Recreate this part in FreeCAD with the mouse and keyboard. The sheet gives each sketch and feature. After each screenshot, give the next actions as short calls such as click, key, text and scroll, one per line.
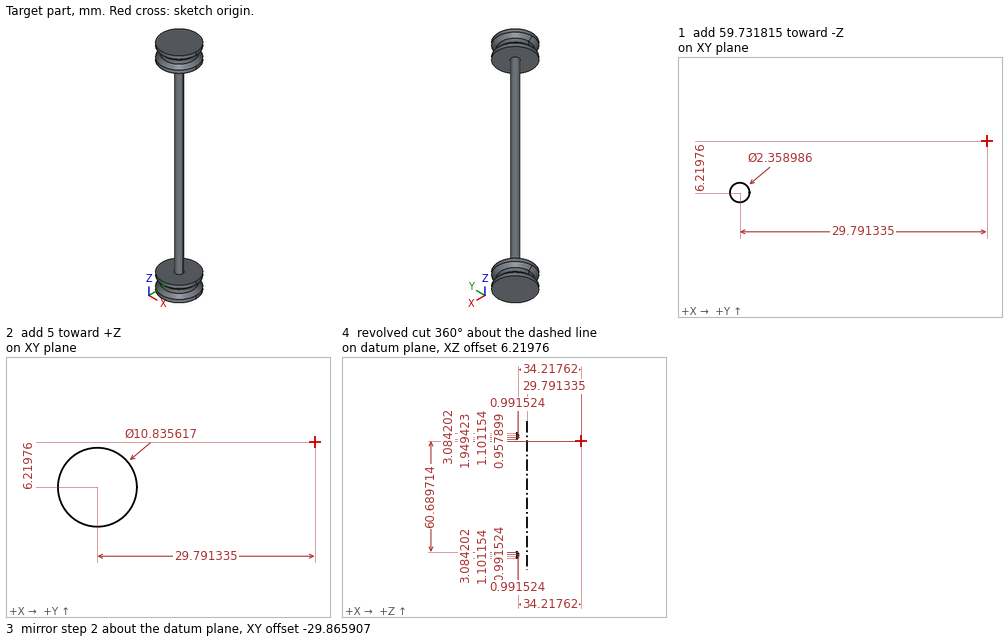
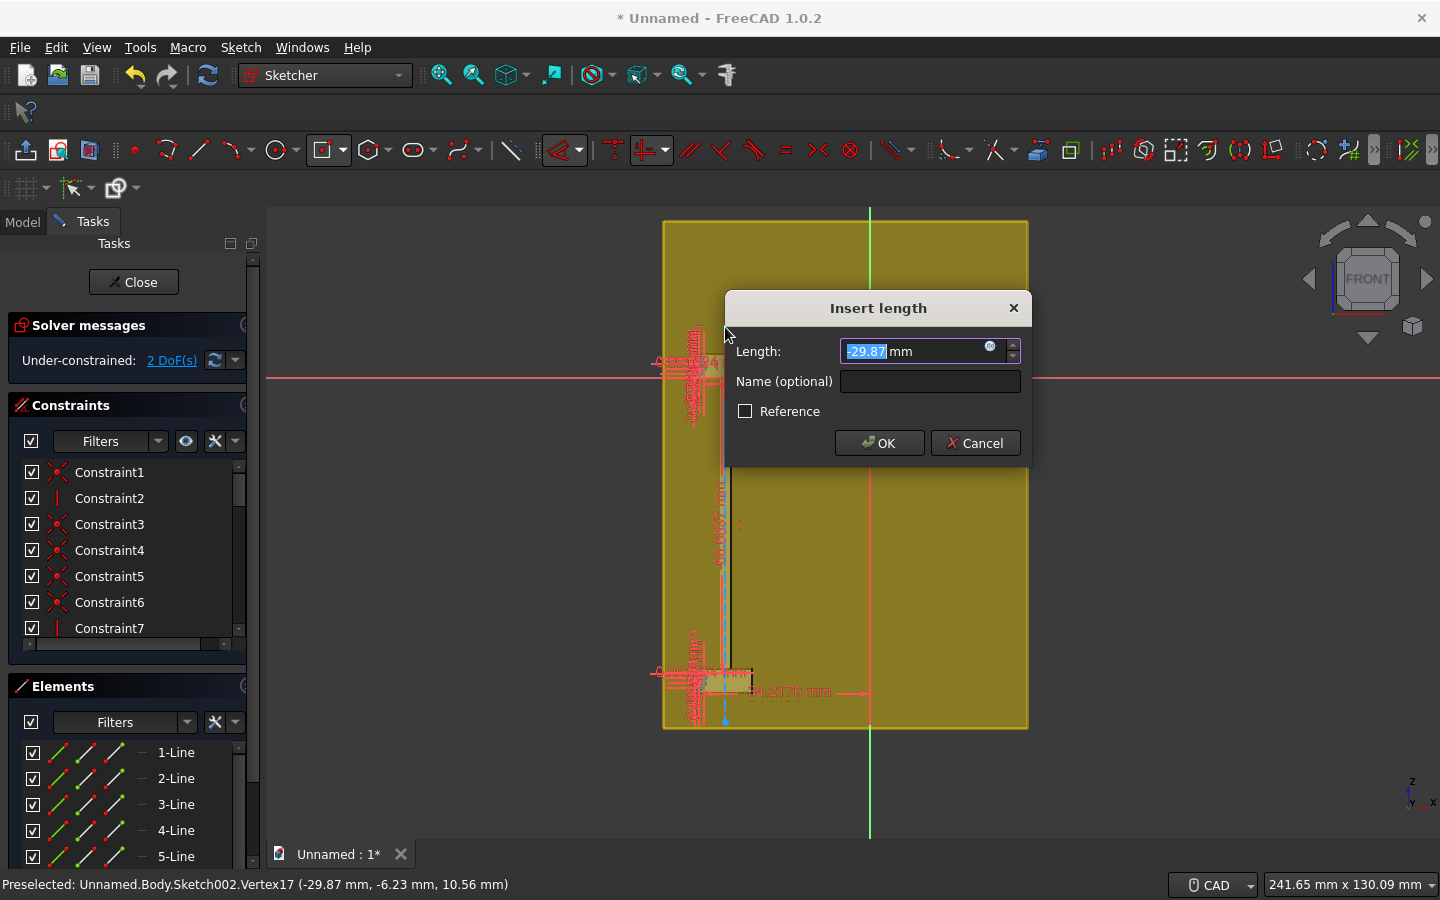
text(-29.791335)
key(Return)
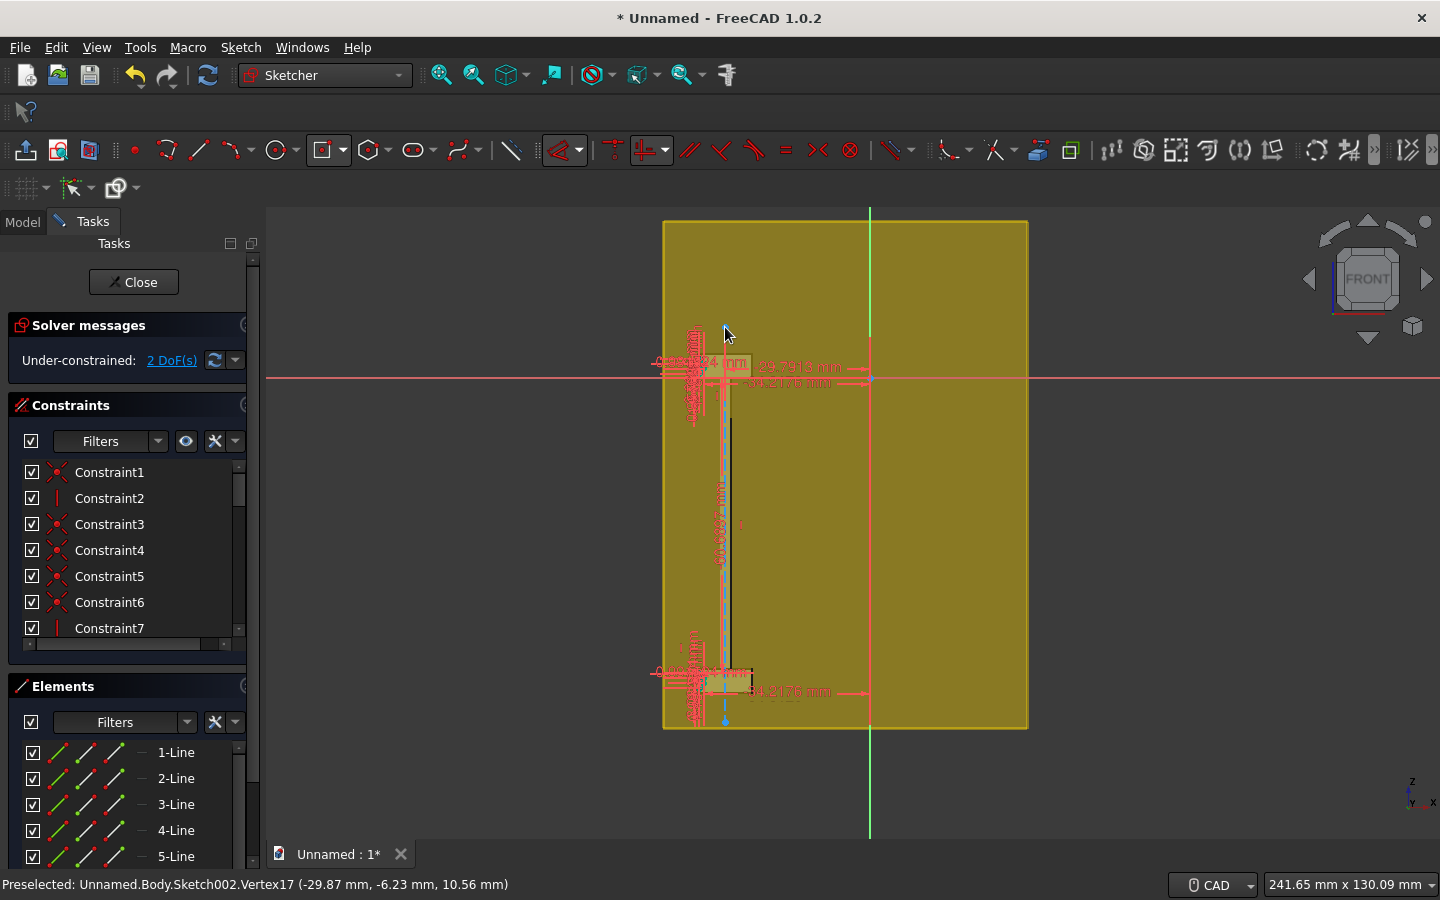
click(134, 282)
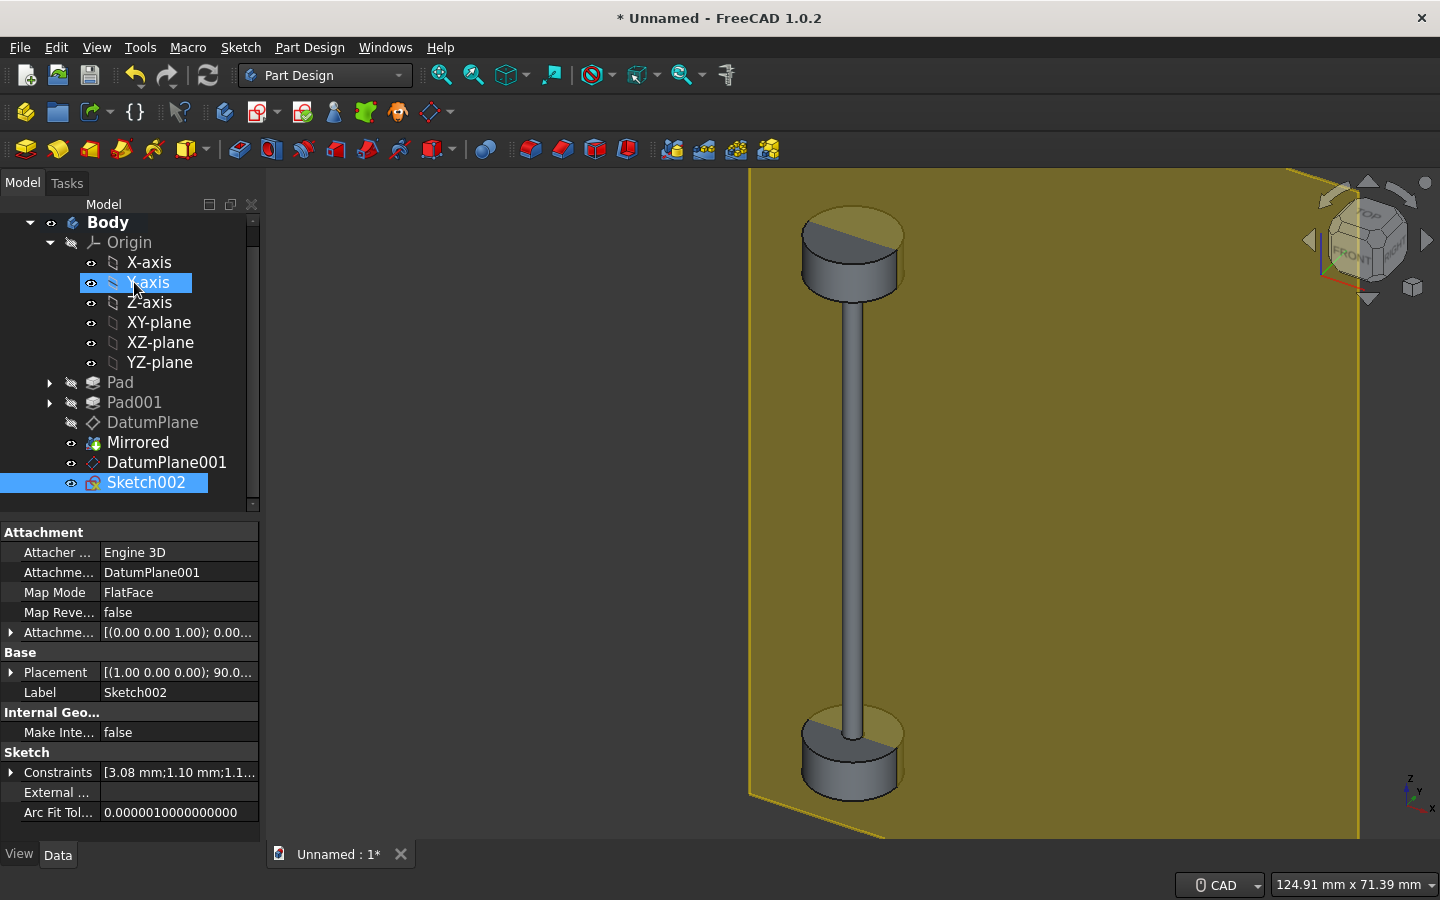
click(304, 150)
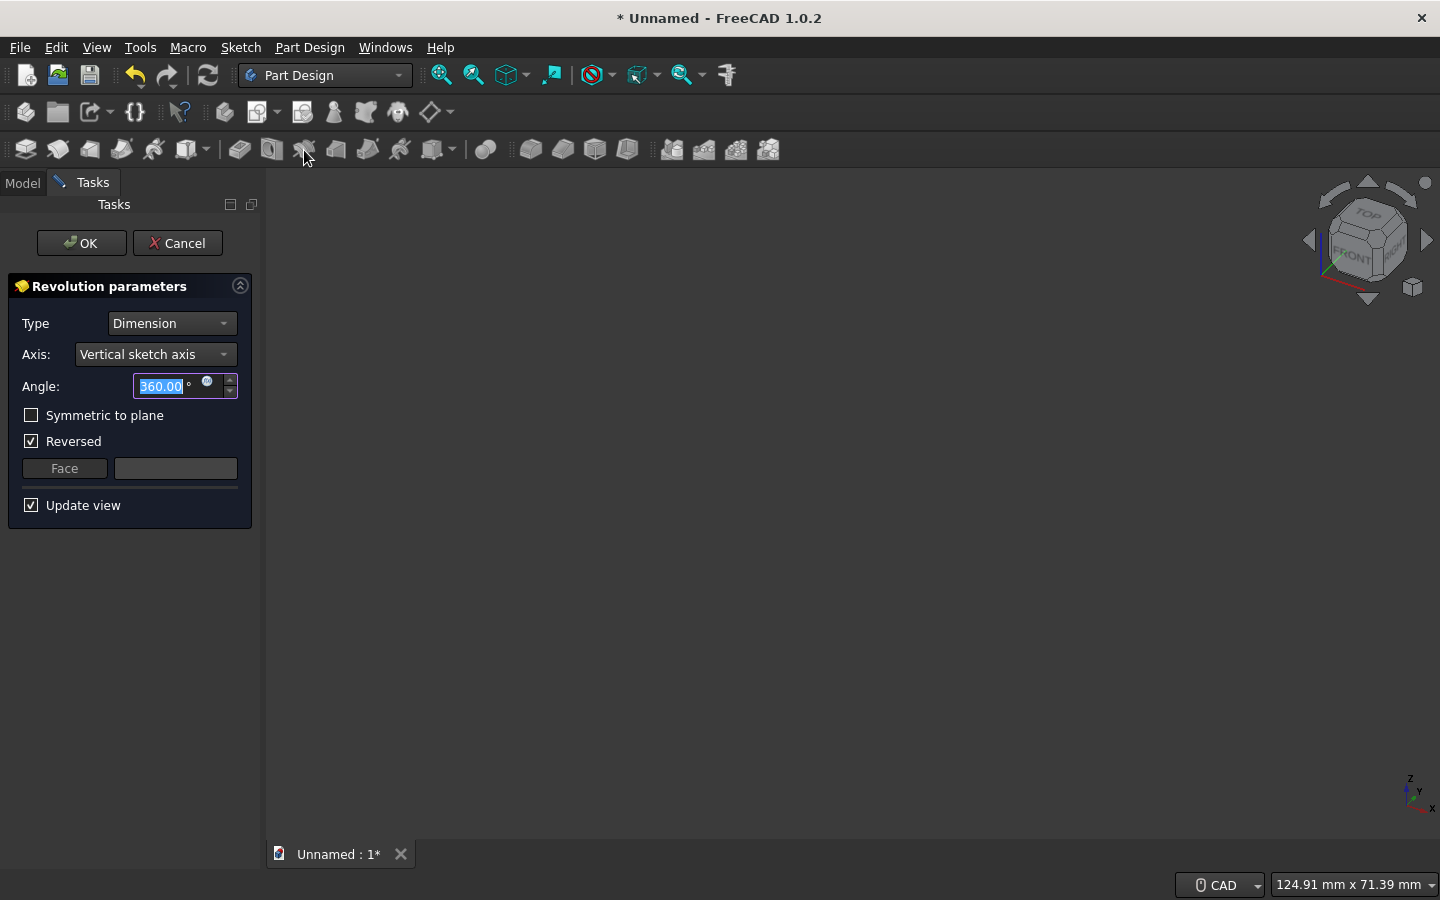
click(156, 354)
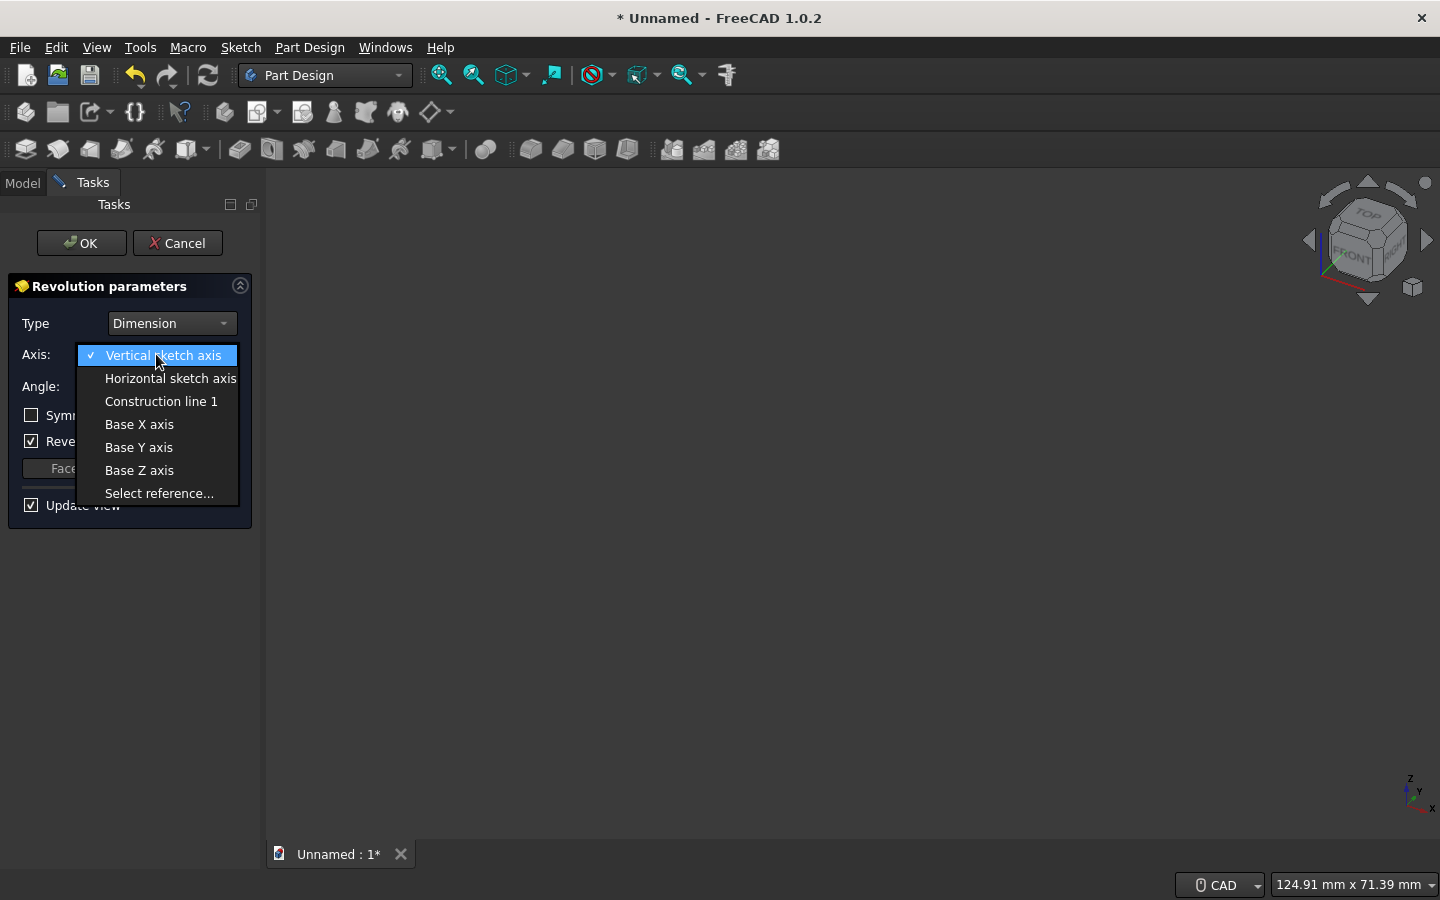
click(156, 402)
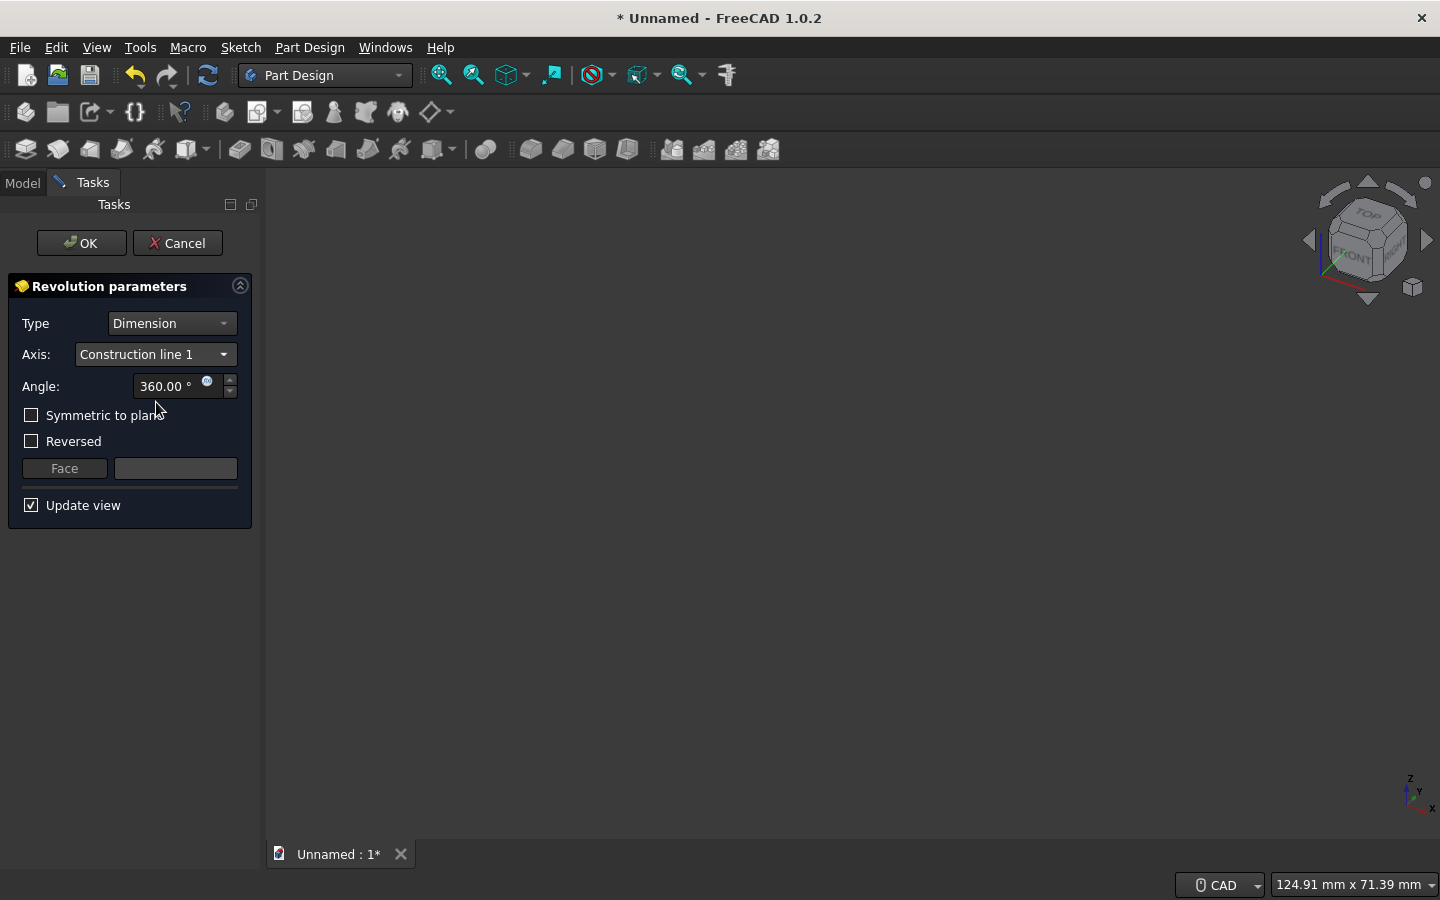
click(82, 243)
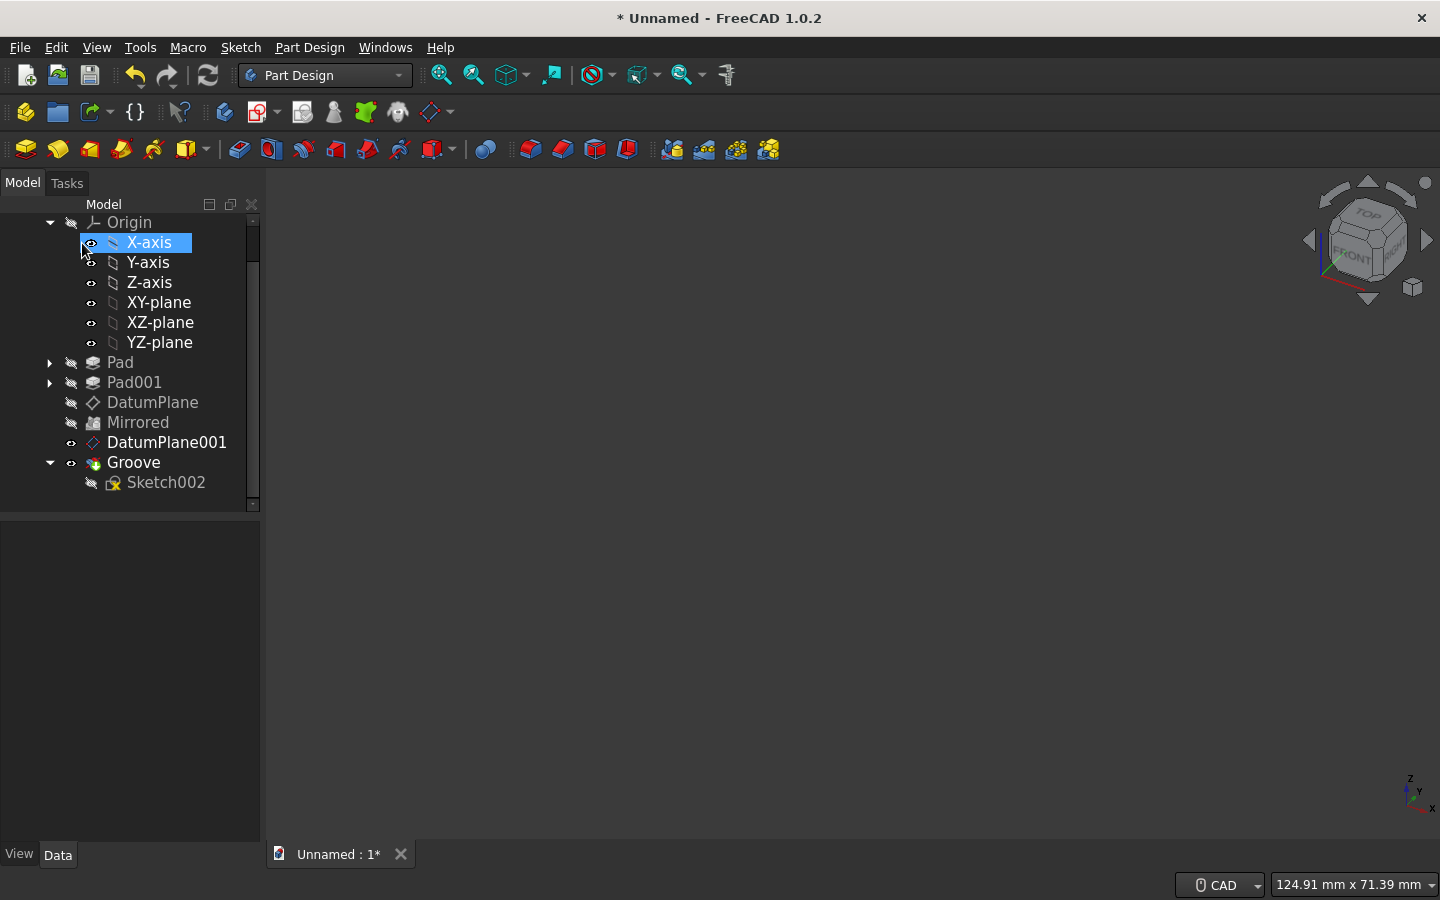
click(116, 443)
key(space)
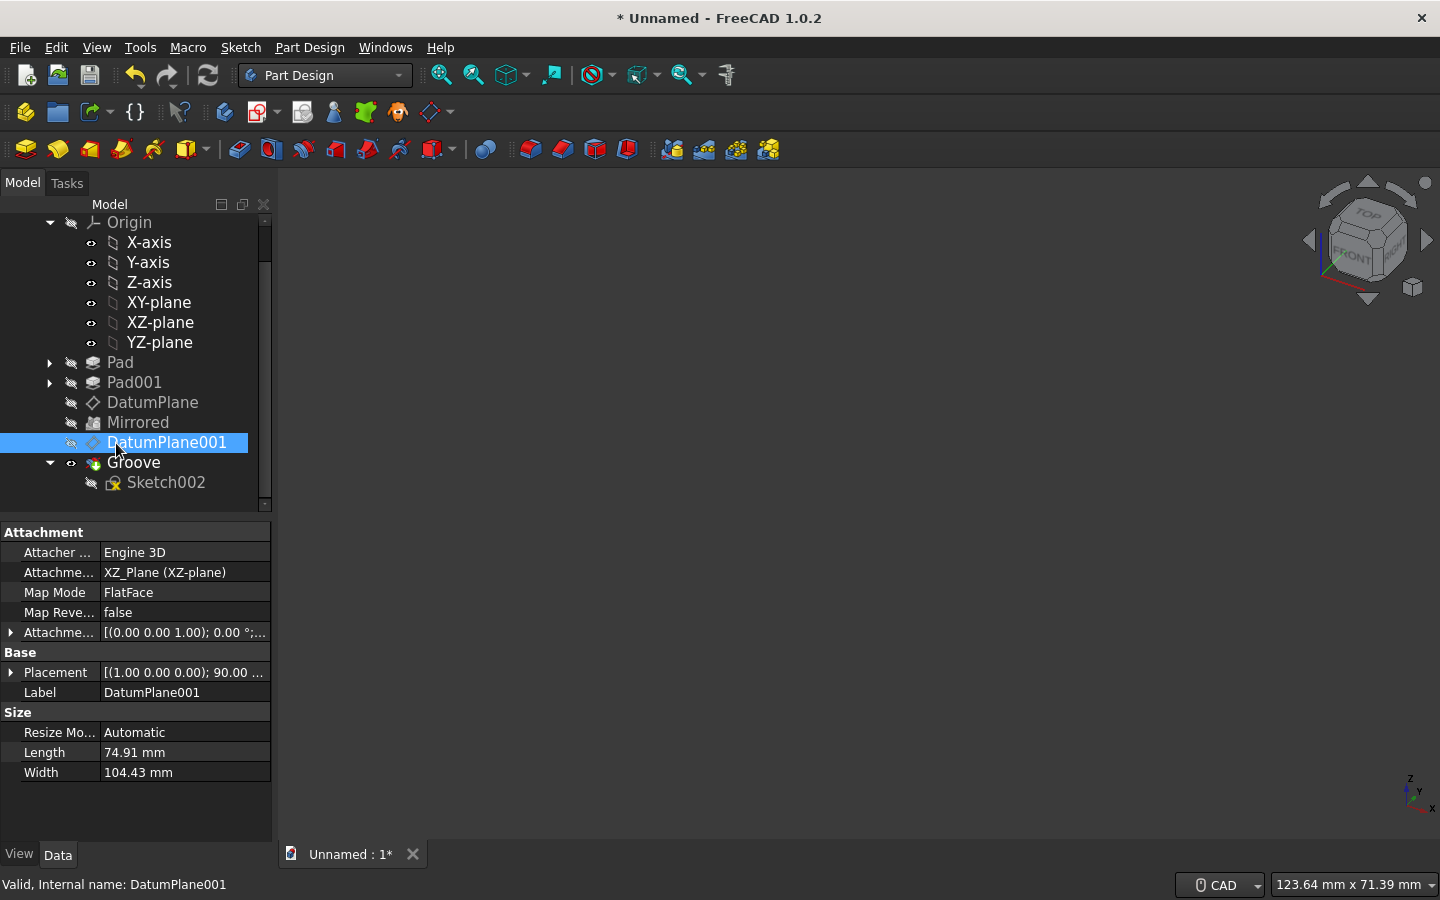
key(0)